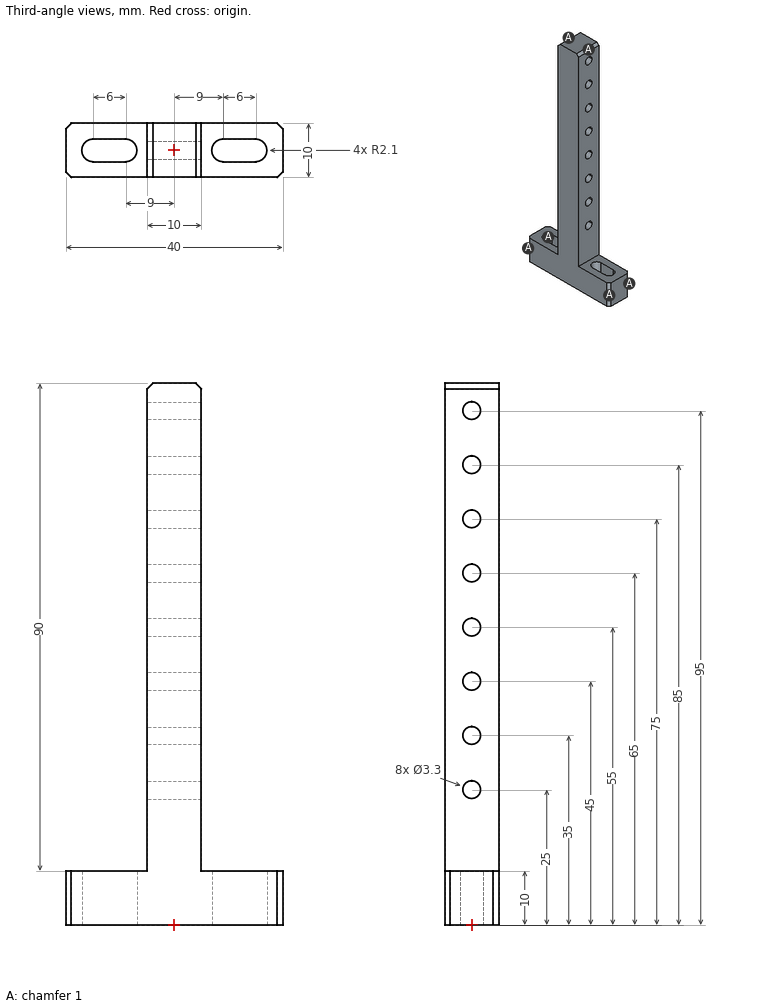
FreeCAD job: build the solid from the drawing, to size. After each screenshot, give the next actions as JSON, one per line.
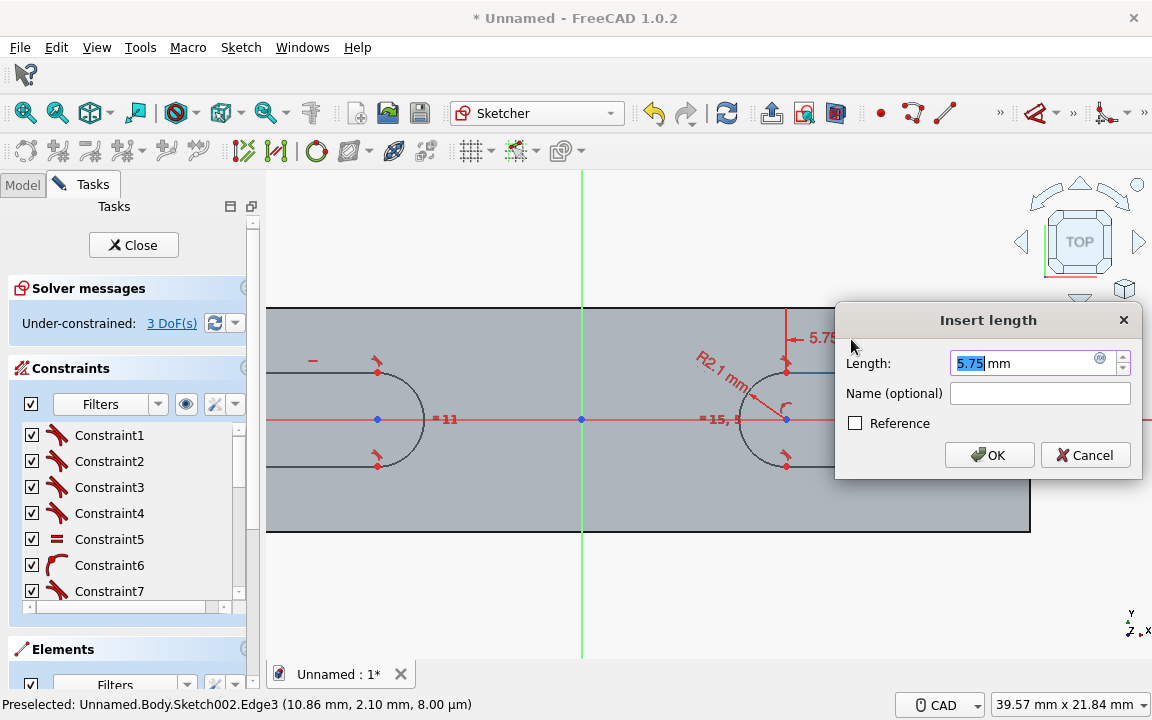
{"action": "type", "text": "6"}
{"action": "key", "text": "Return"}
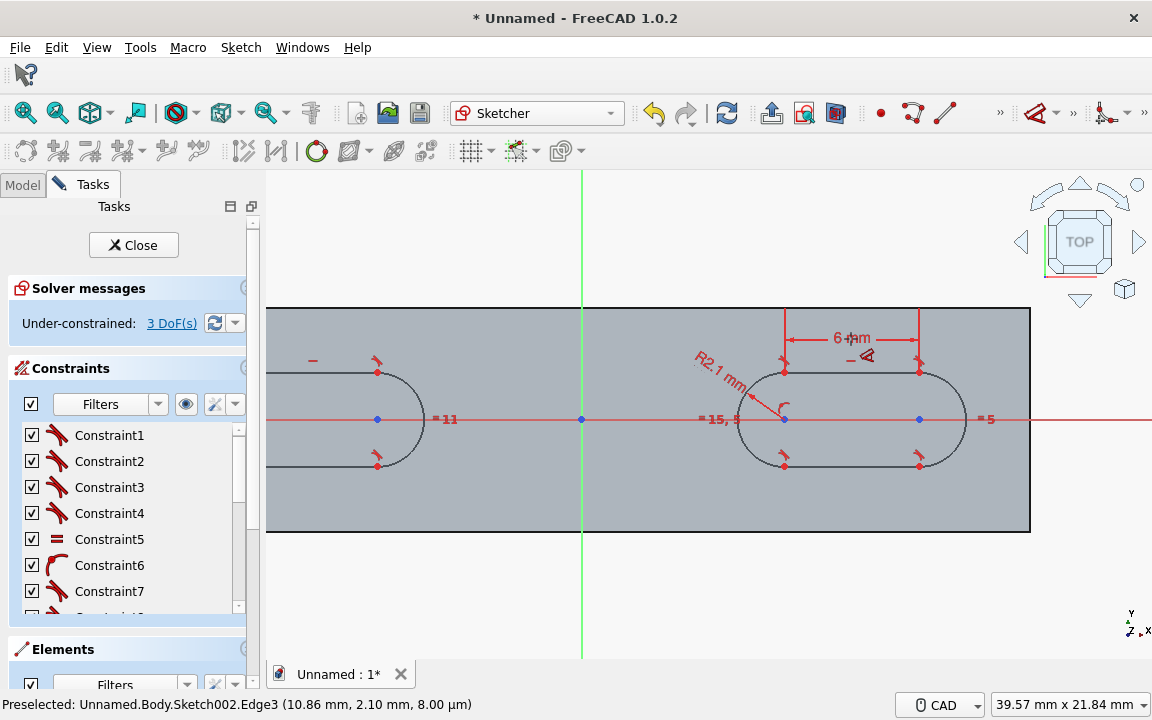
{"action": "left_click", "coordinate": [339, 373]}
{"action": "left_click", "coordinate": [336, 339]}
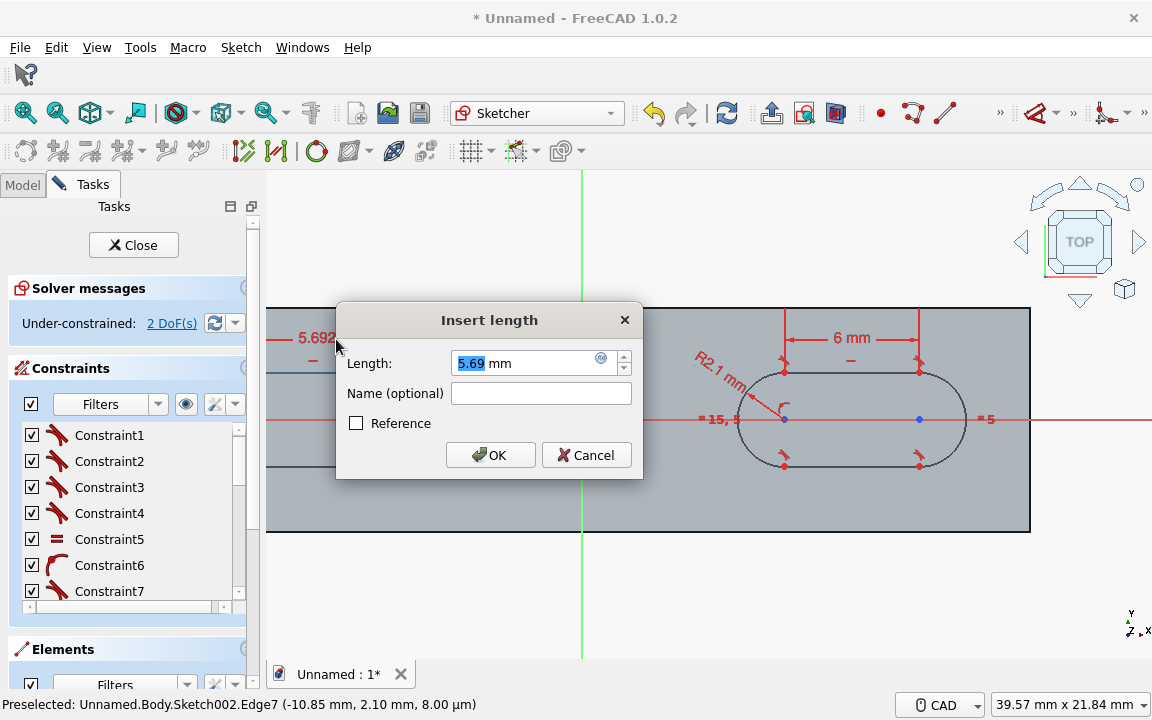
{"action": "type", "text": "6"}
{"action": "key", "text": "Return"}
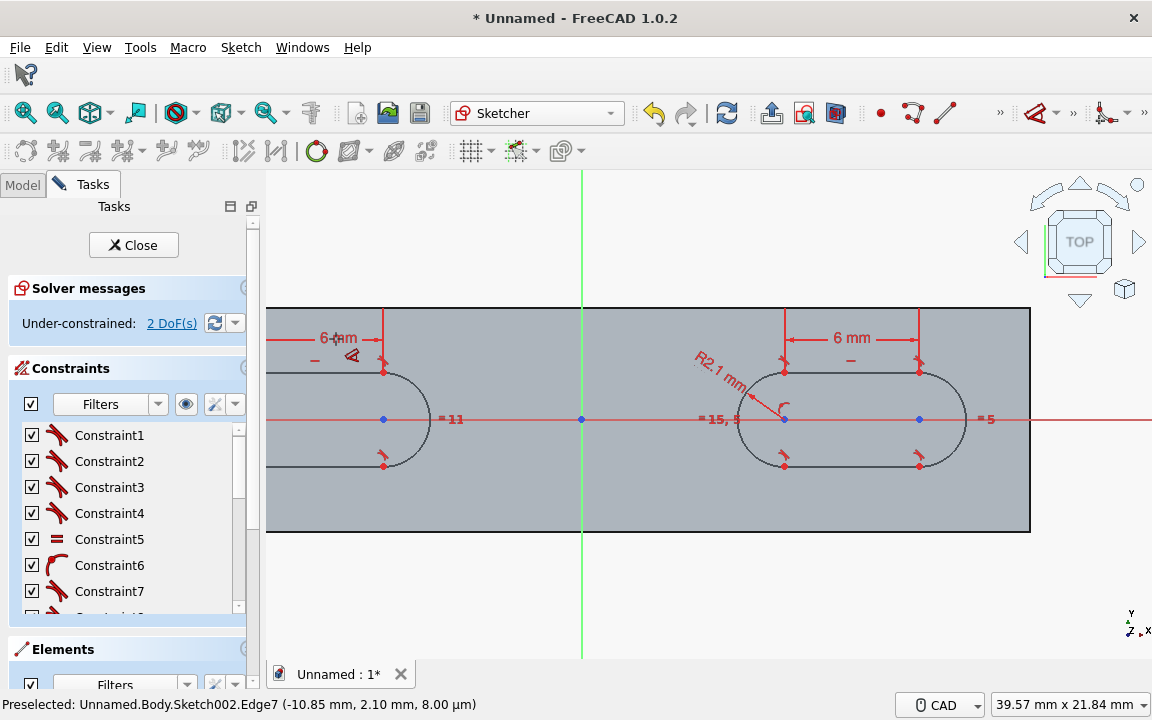
{"action": "left_click", "coordinate": [785, 373]}
{"action": "left_click", "coordinate": [683, 339]}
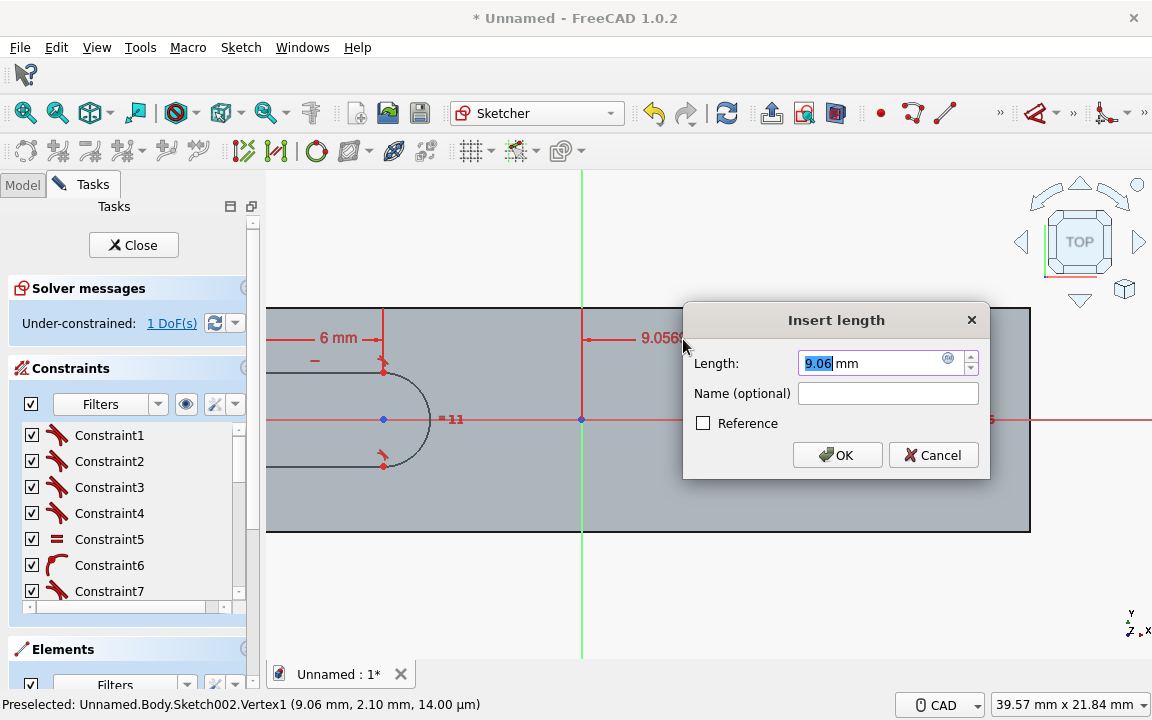
{"action": "type", "text": "9"}
{"action": "key", "text": "Return"}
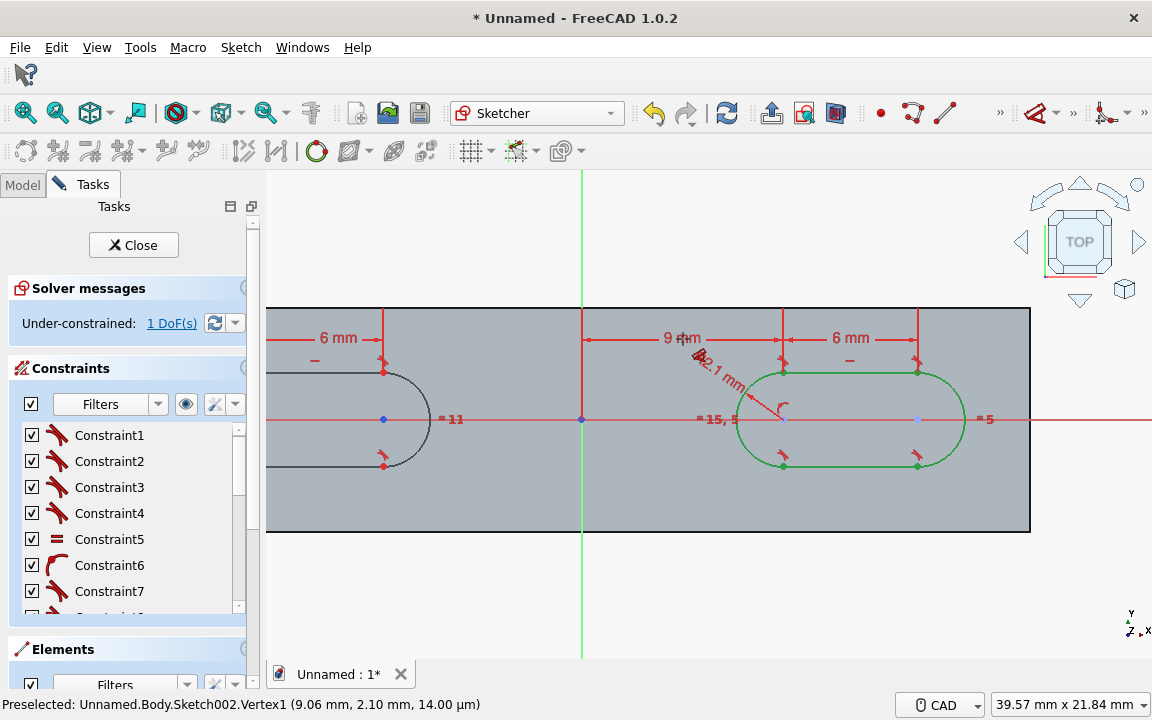
{"action": "left_click", "coordinate": [383, 467]}
{"action": "left_click", "coordinate": [482, 501]}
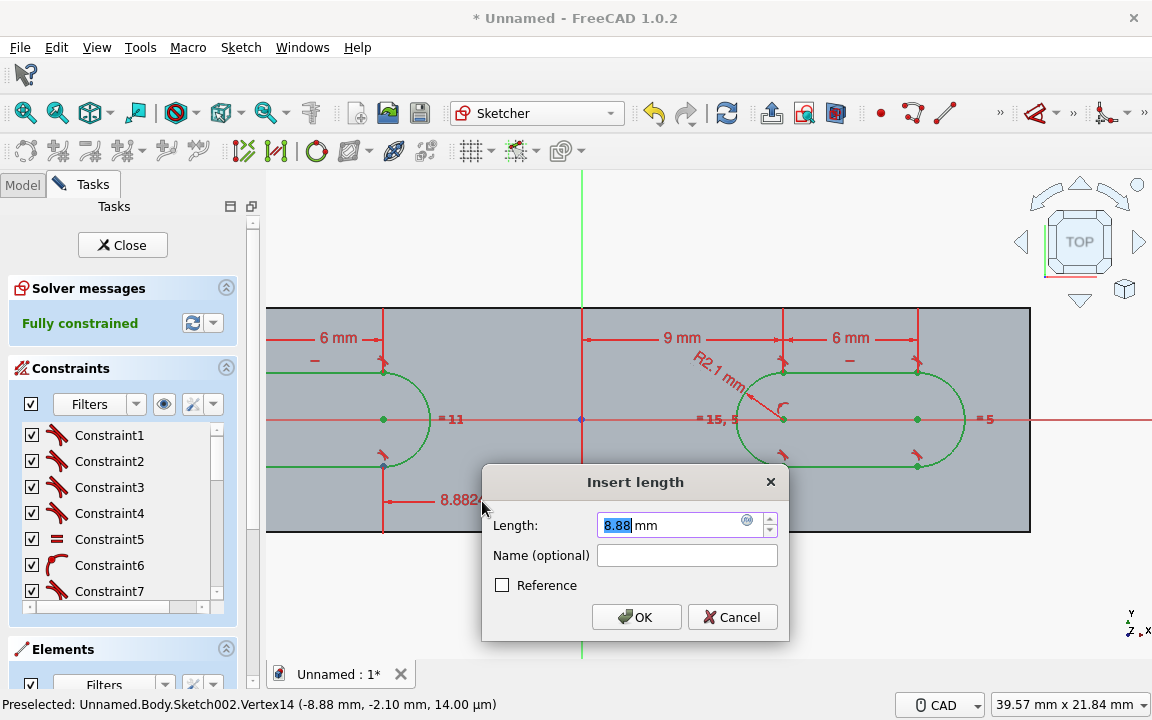
{"action": "type", "text": "9"}
{"action": "key", "text": "Return"}
{"action": "key", "text": "Escape"}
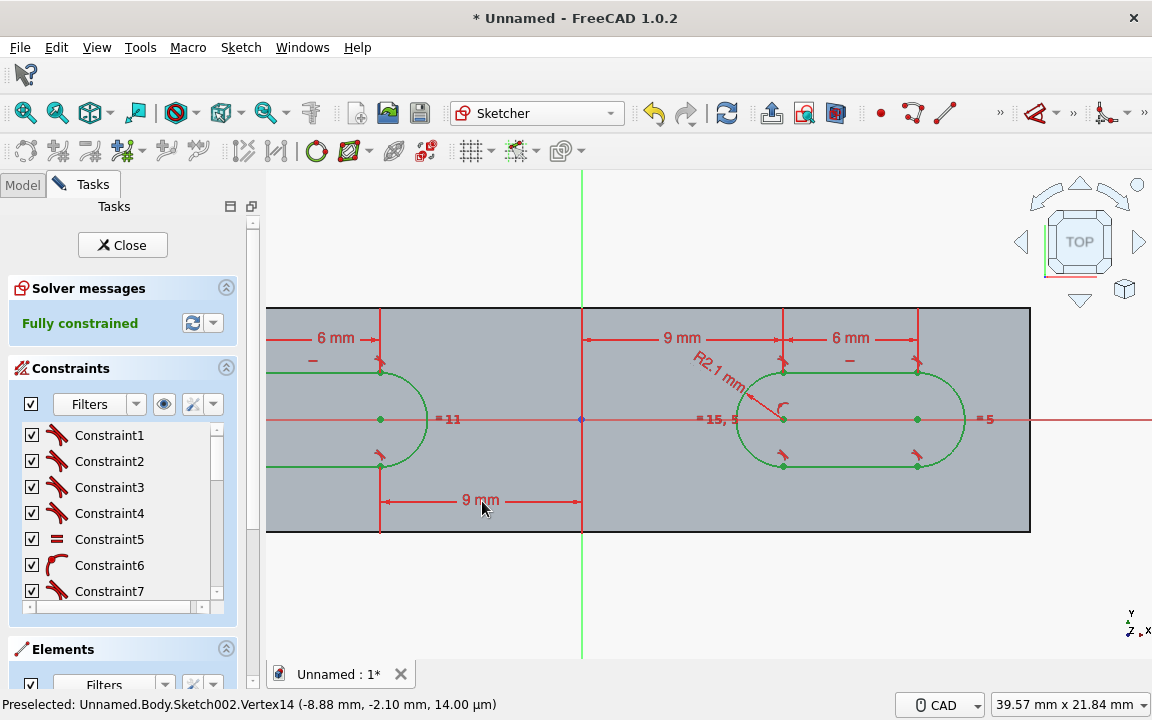
{"action": "left_click", "coordinate": [123, 245]}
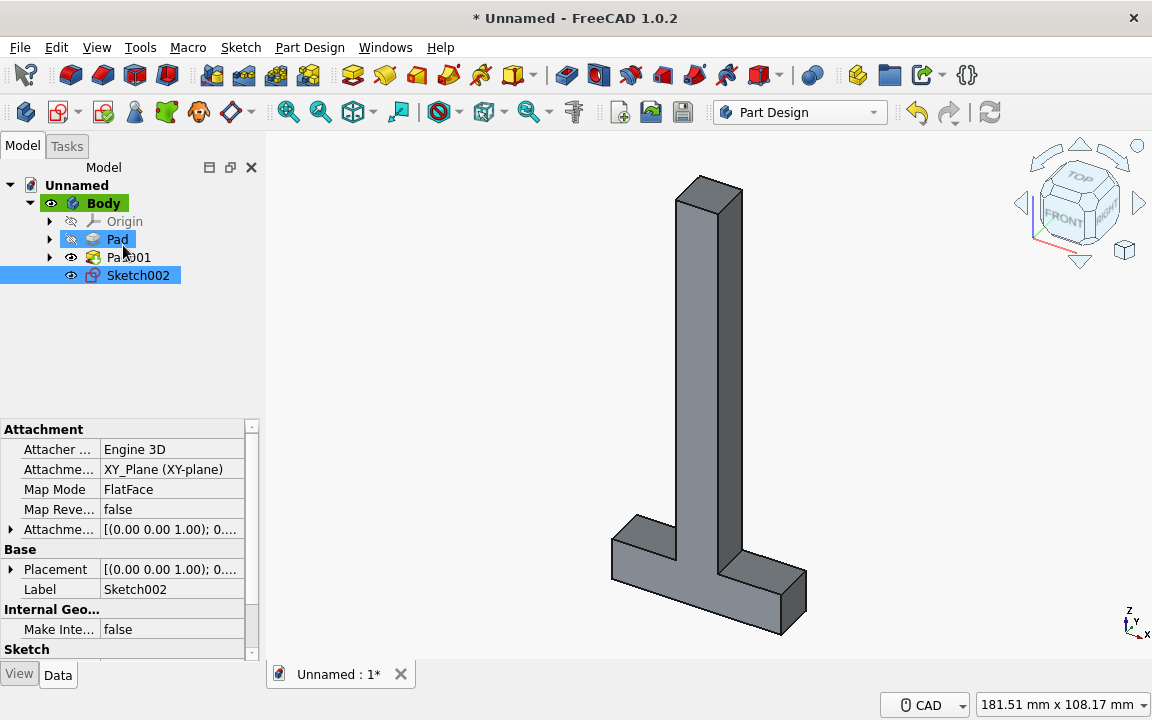
{"action": "left_click", "coordinate": [568, 76]}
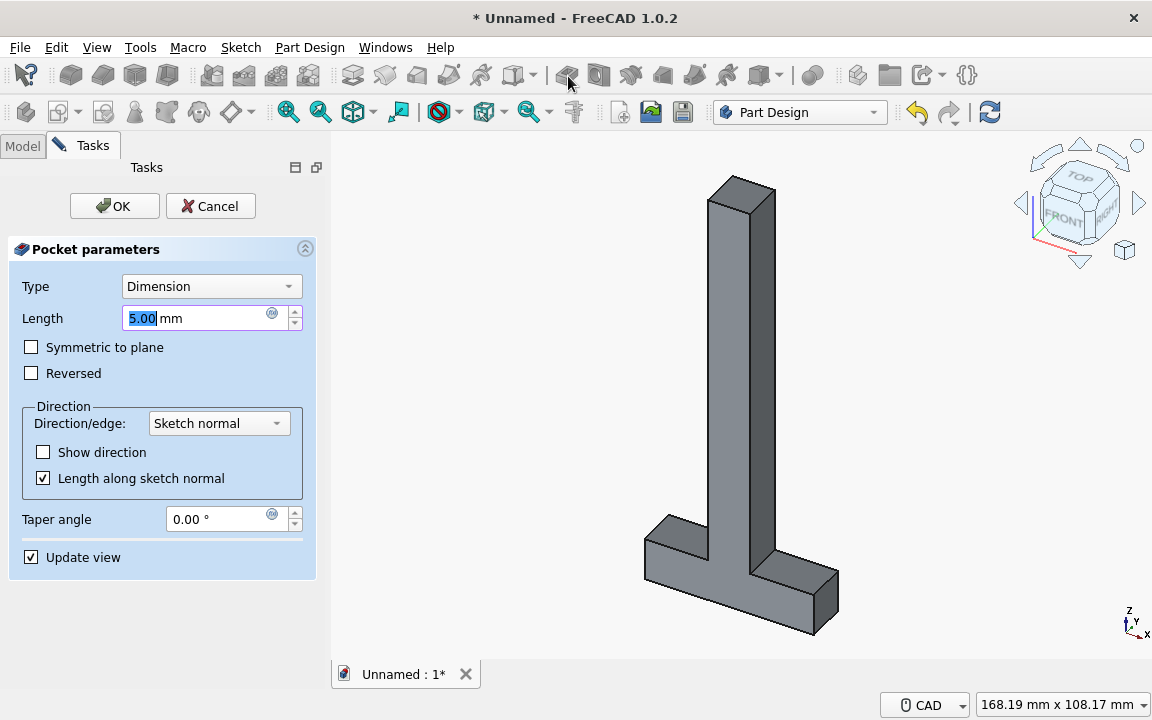
{"action": "left_click", "coordinate": [212, 286]}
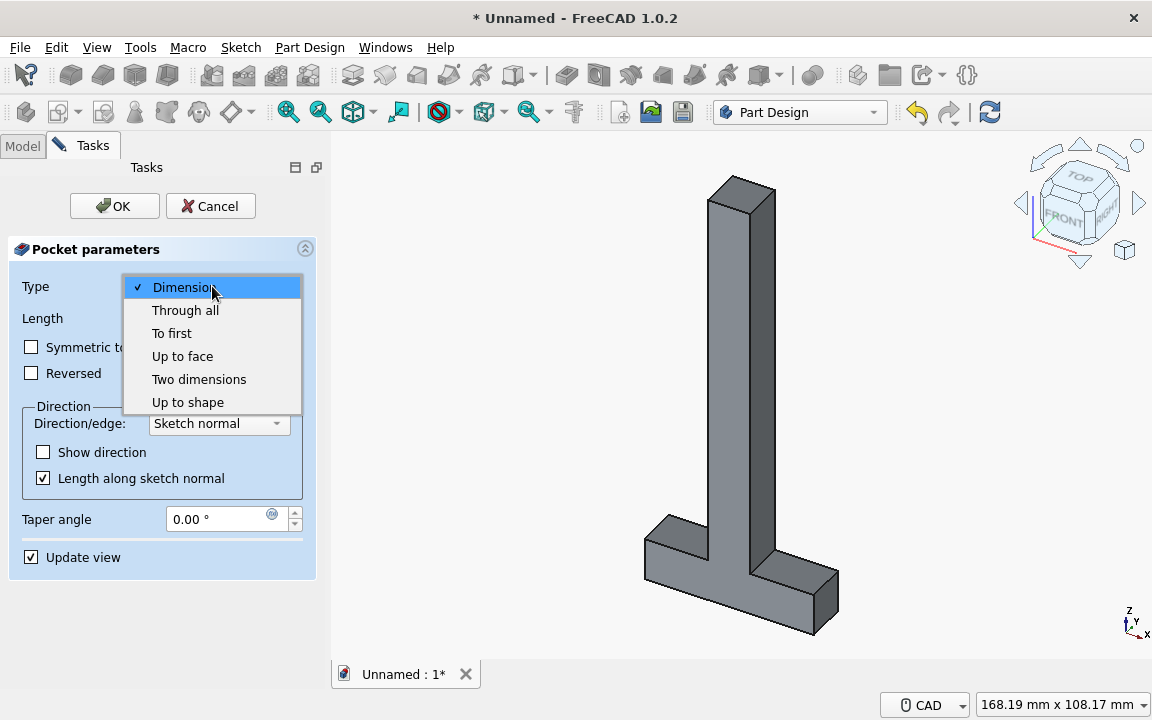
{"action": "left_click", "coordinate": [212, 310]}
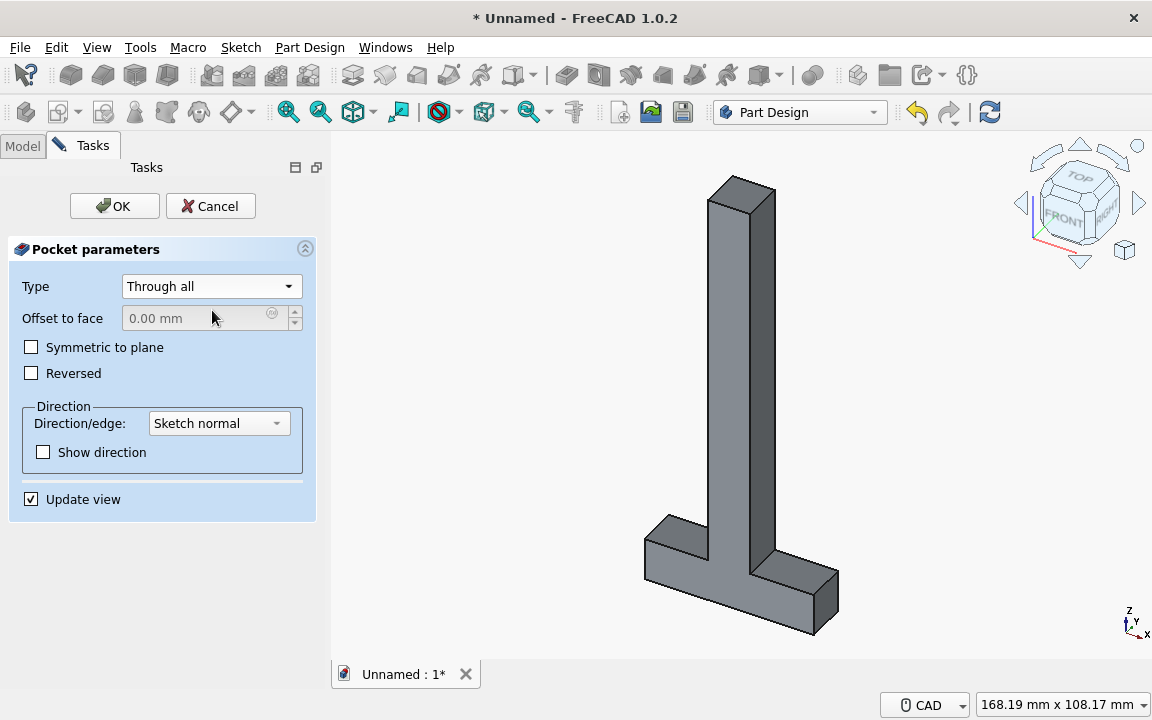
{"action": "left_click", "coordinate": [30, 373]}